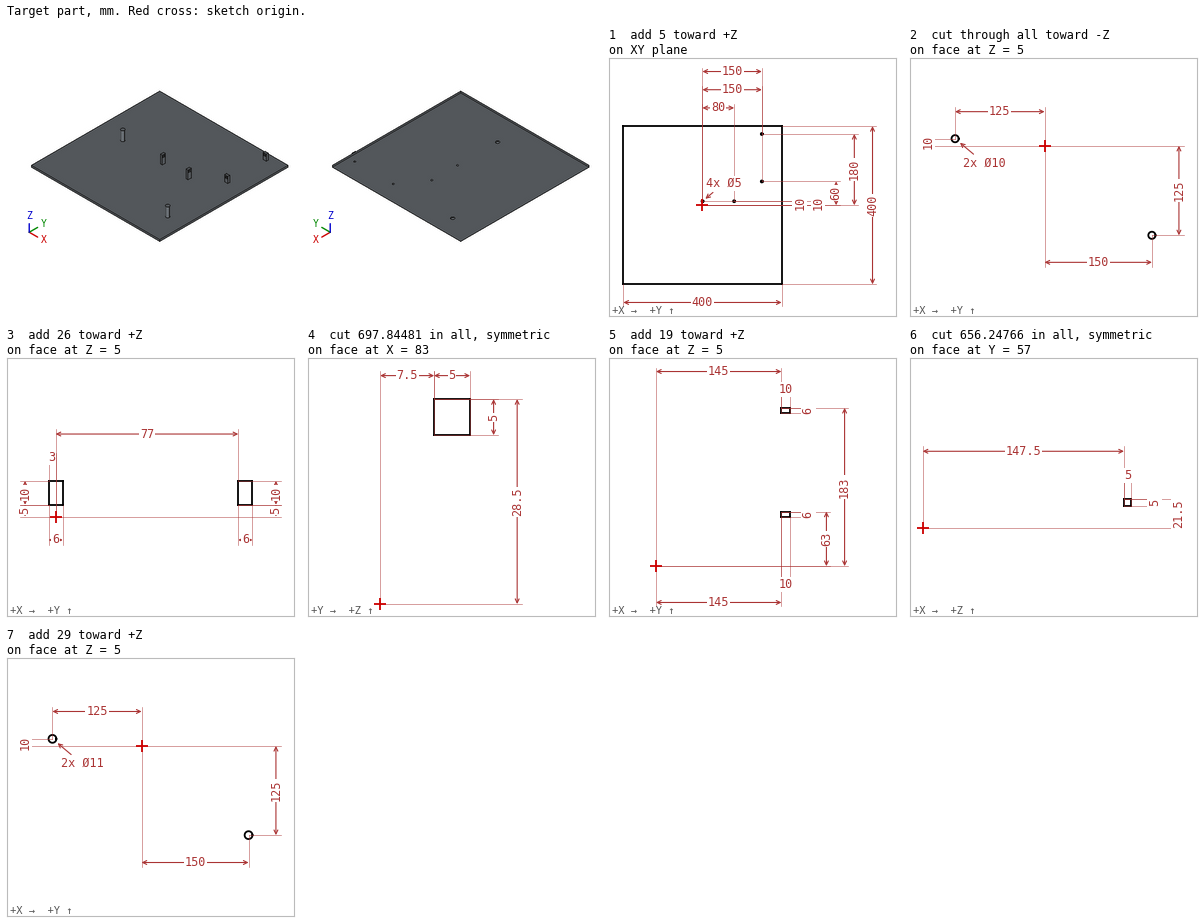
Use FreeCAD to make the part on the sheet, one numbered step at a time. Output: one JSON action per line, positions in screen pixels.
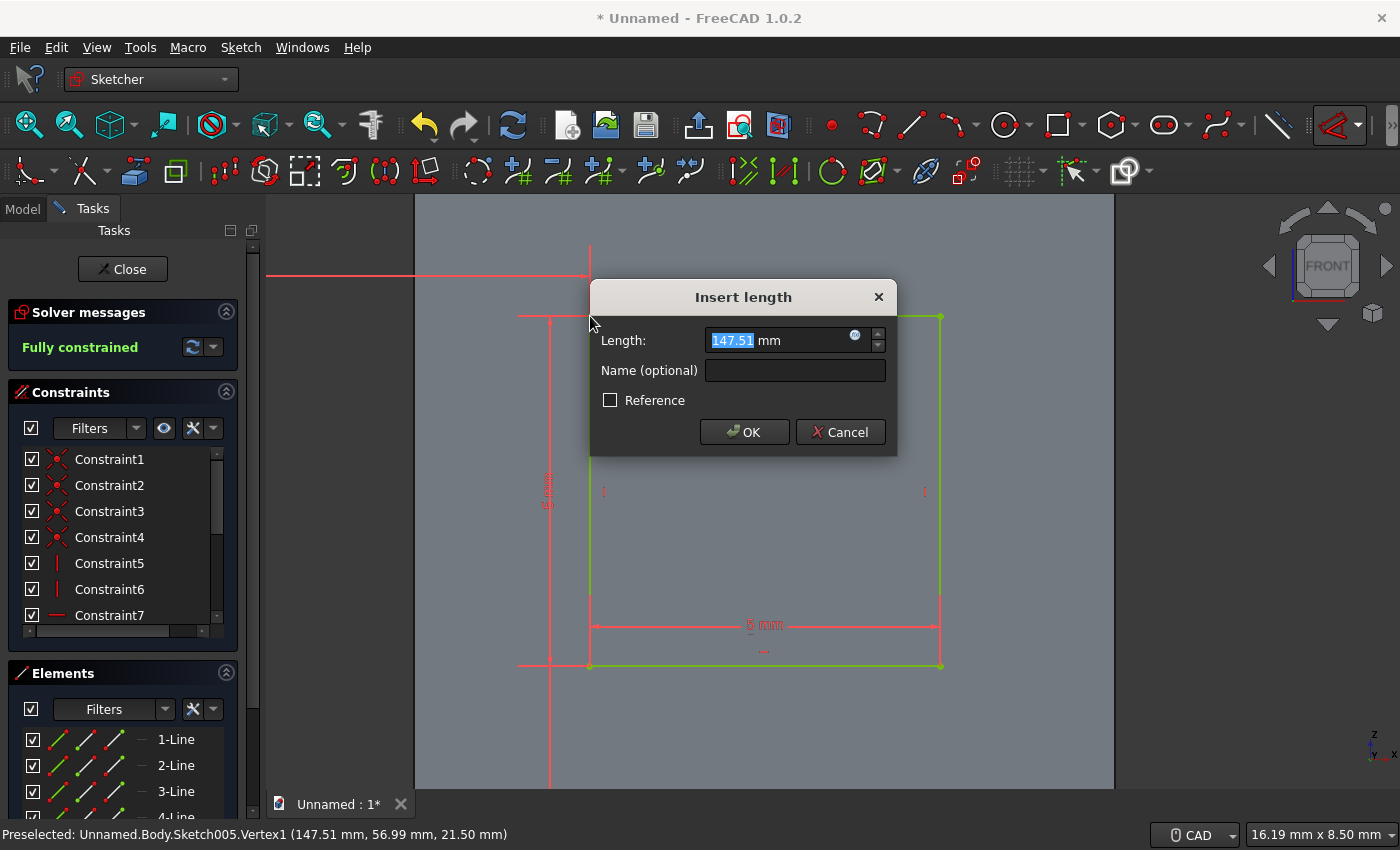
{"action": "type", "text": "147.5"}
{"action": "key", "text": "Return"}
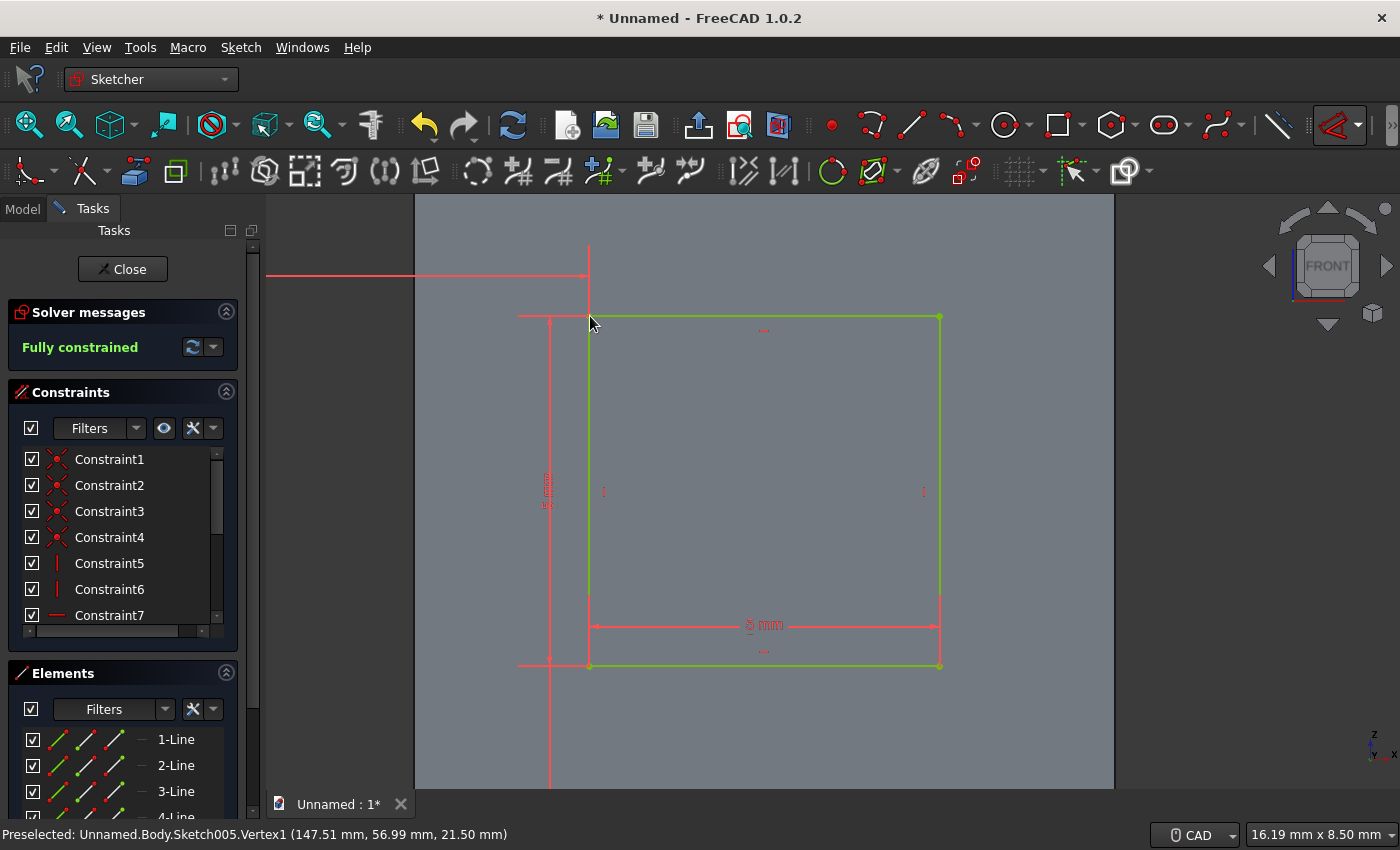
{"action": "left_click", "coordinate": [123, 269]}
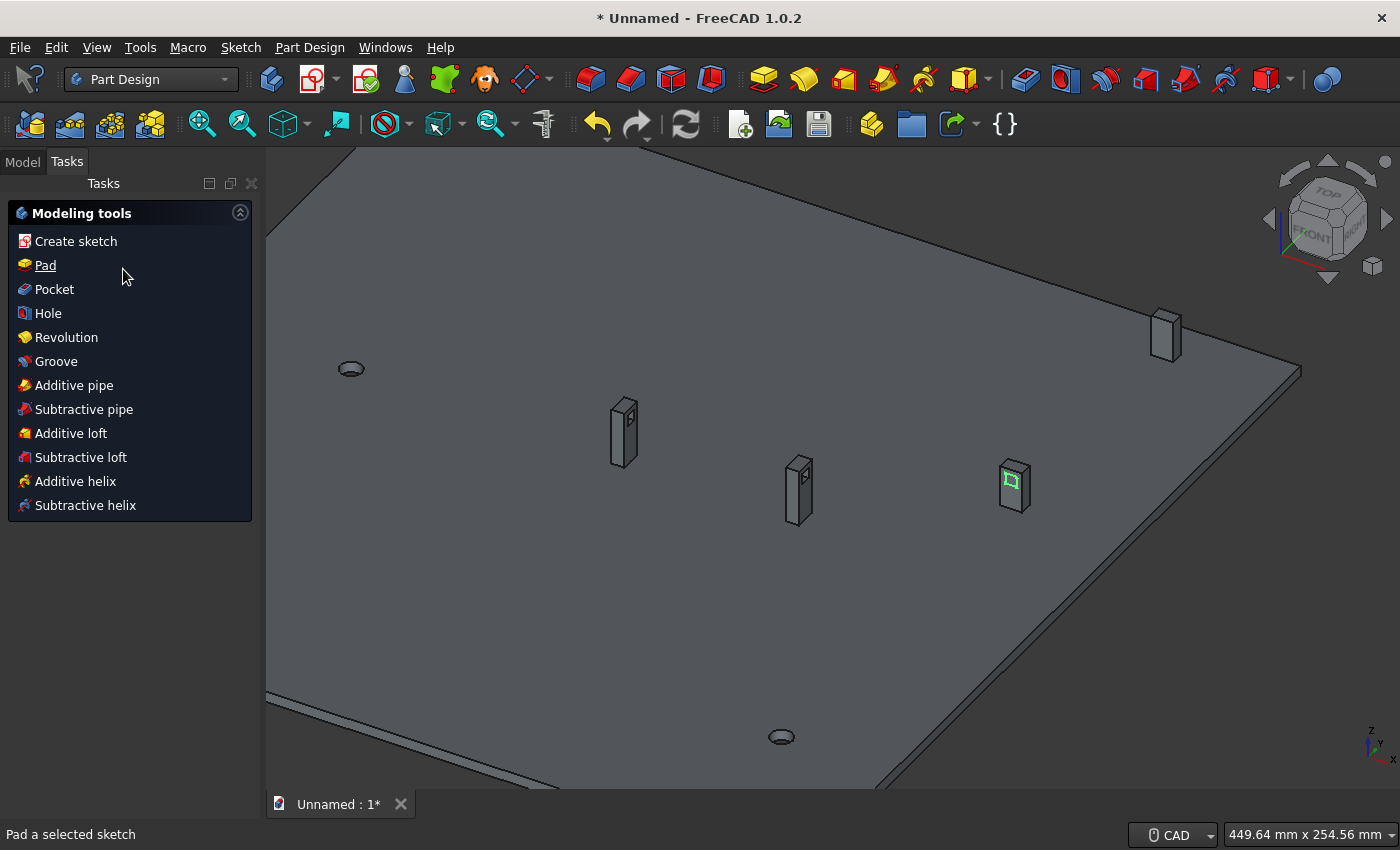
{"action": "left_click", "coordinate": [1026, 80]}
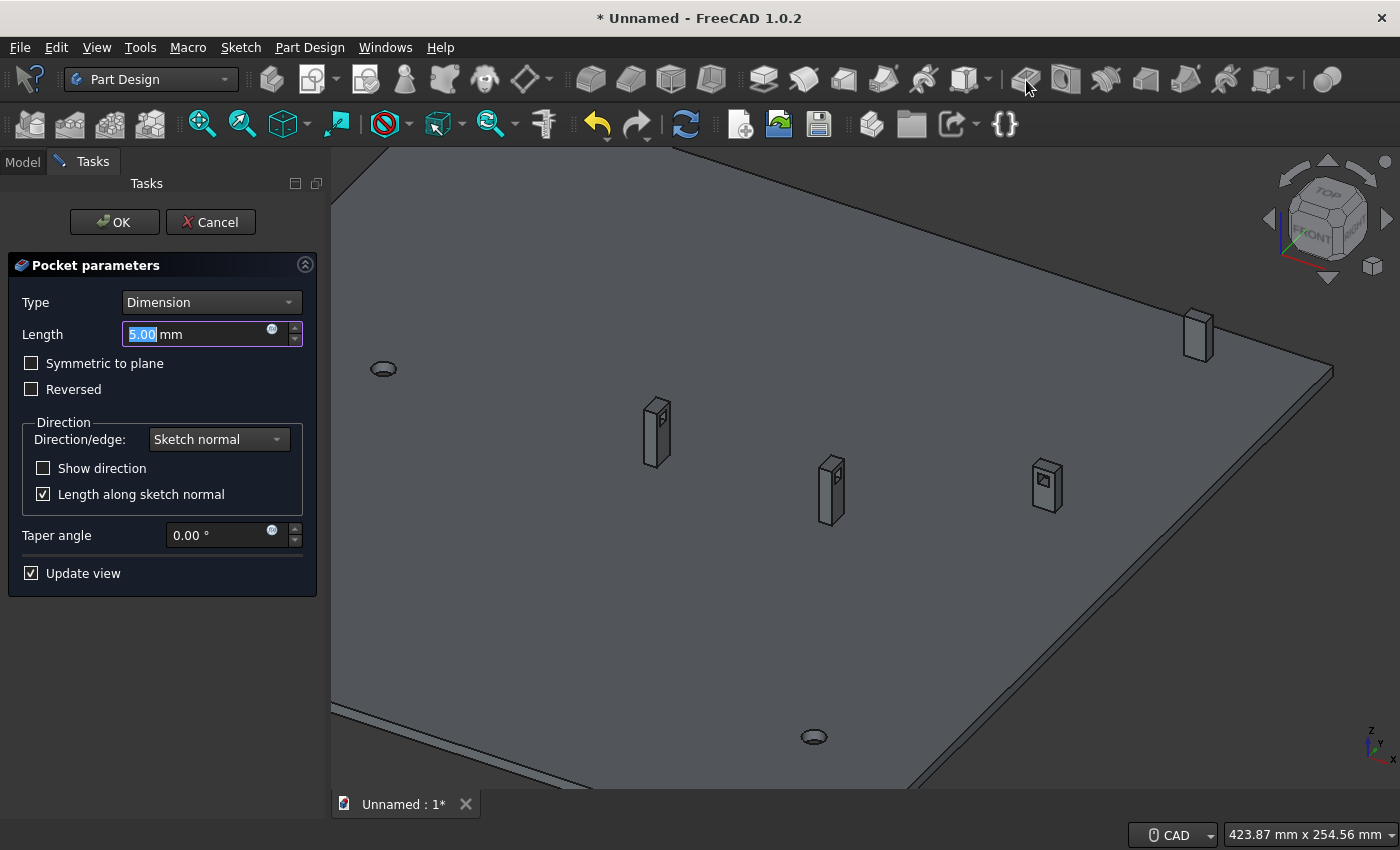
{"action": "type", "text": "656.24766"}
{"action": "key", "text": "Tab"}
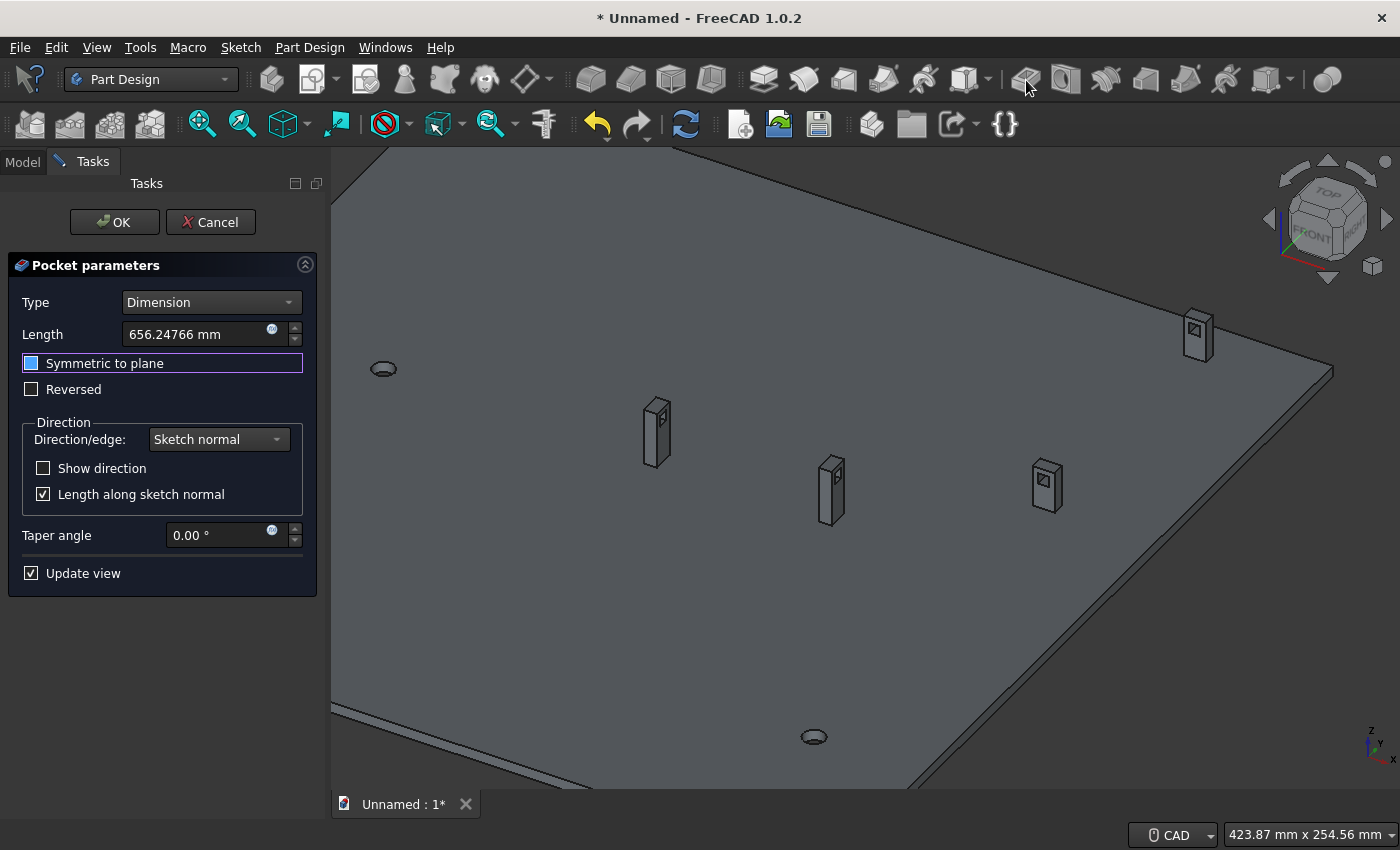
{"action": "left_click", "coordinate": [30, 363]}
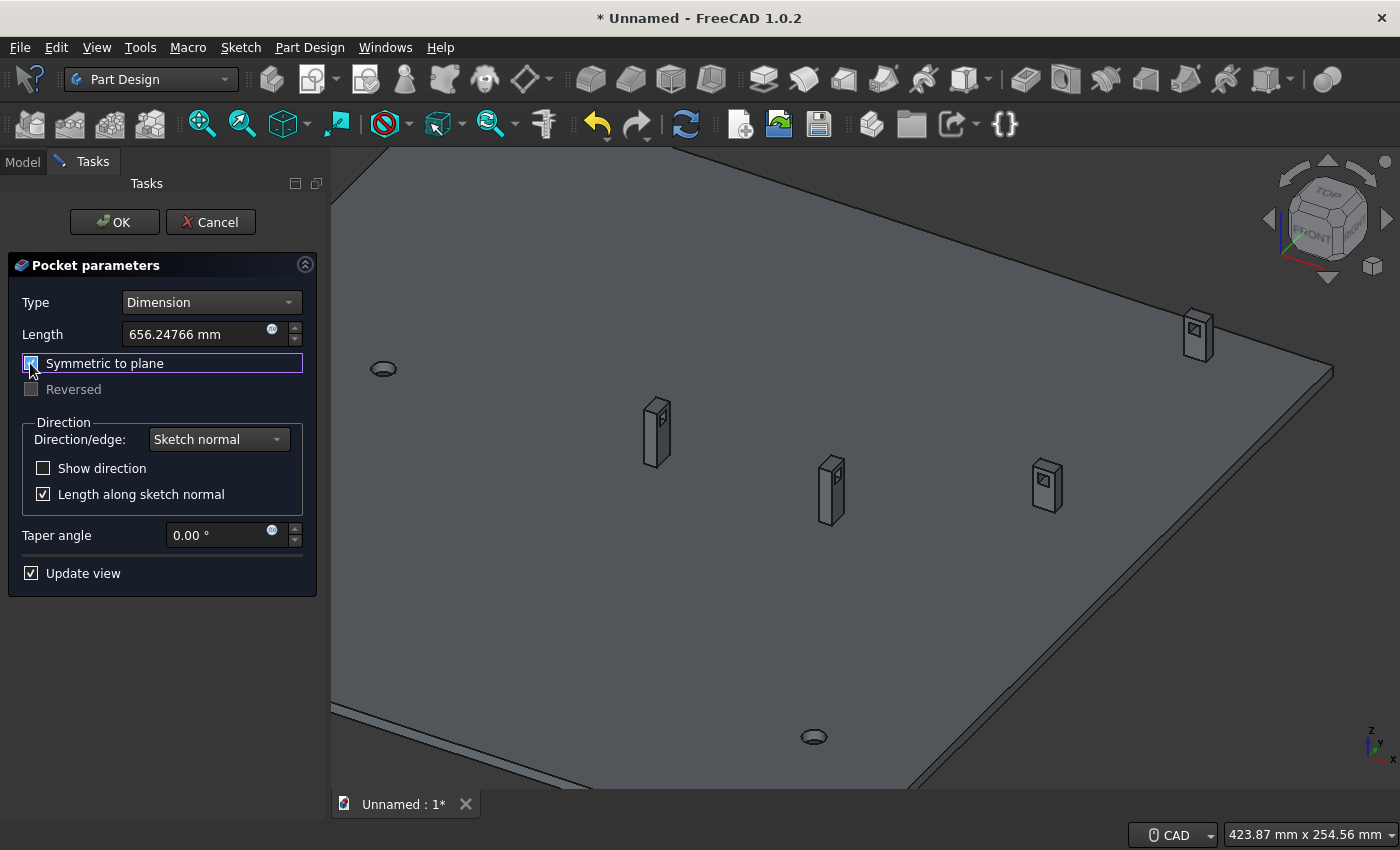
{"action": "left_click", "coordinate": [115, 222]}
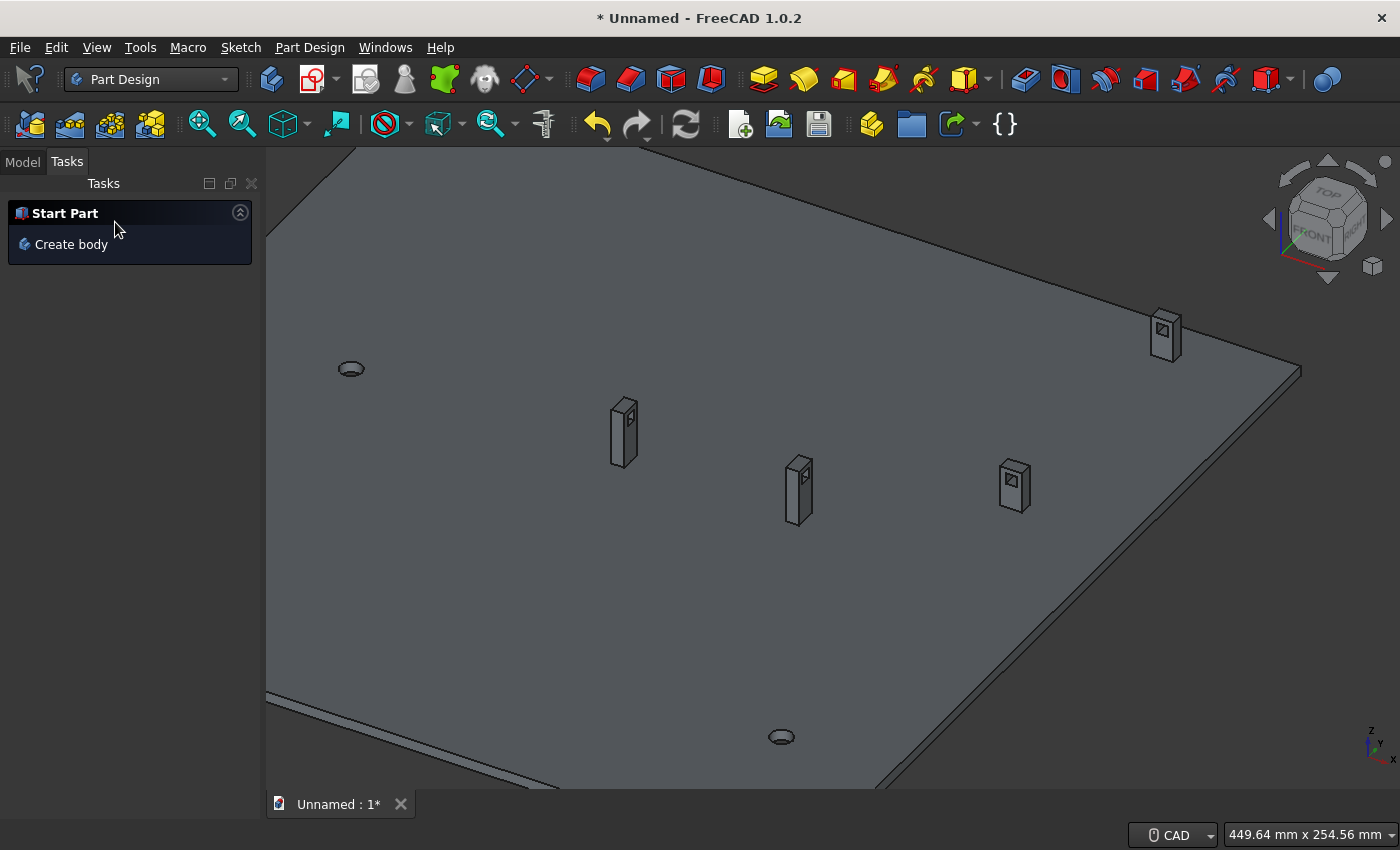
{"action": "key", "text": "v f"}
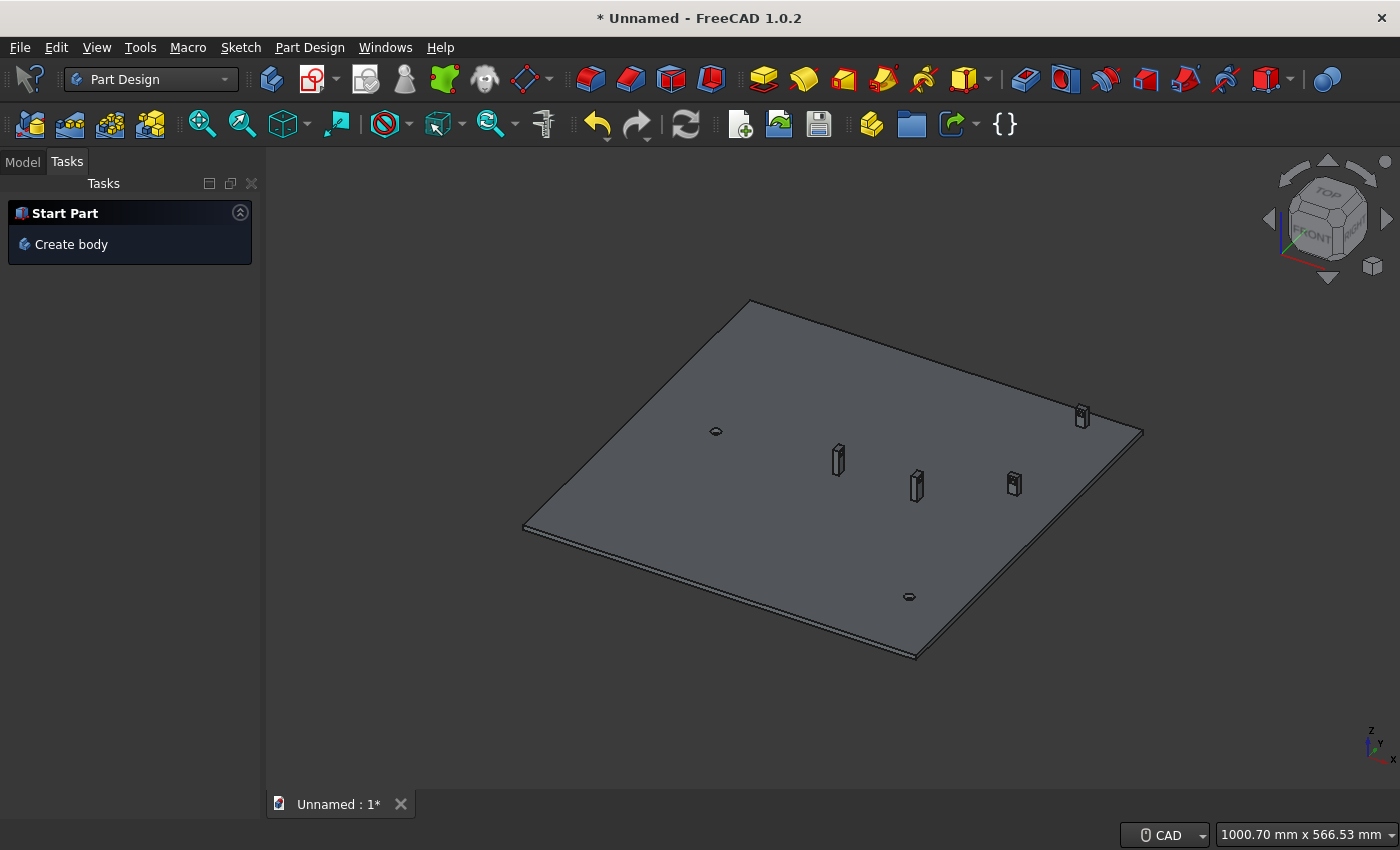
{"action": "left_click", "coordinate": [954, 431]}